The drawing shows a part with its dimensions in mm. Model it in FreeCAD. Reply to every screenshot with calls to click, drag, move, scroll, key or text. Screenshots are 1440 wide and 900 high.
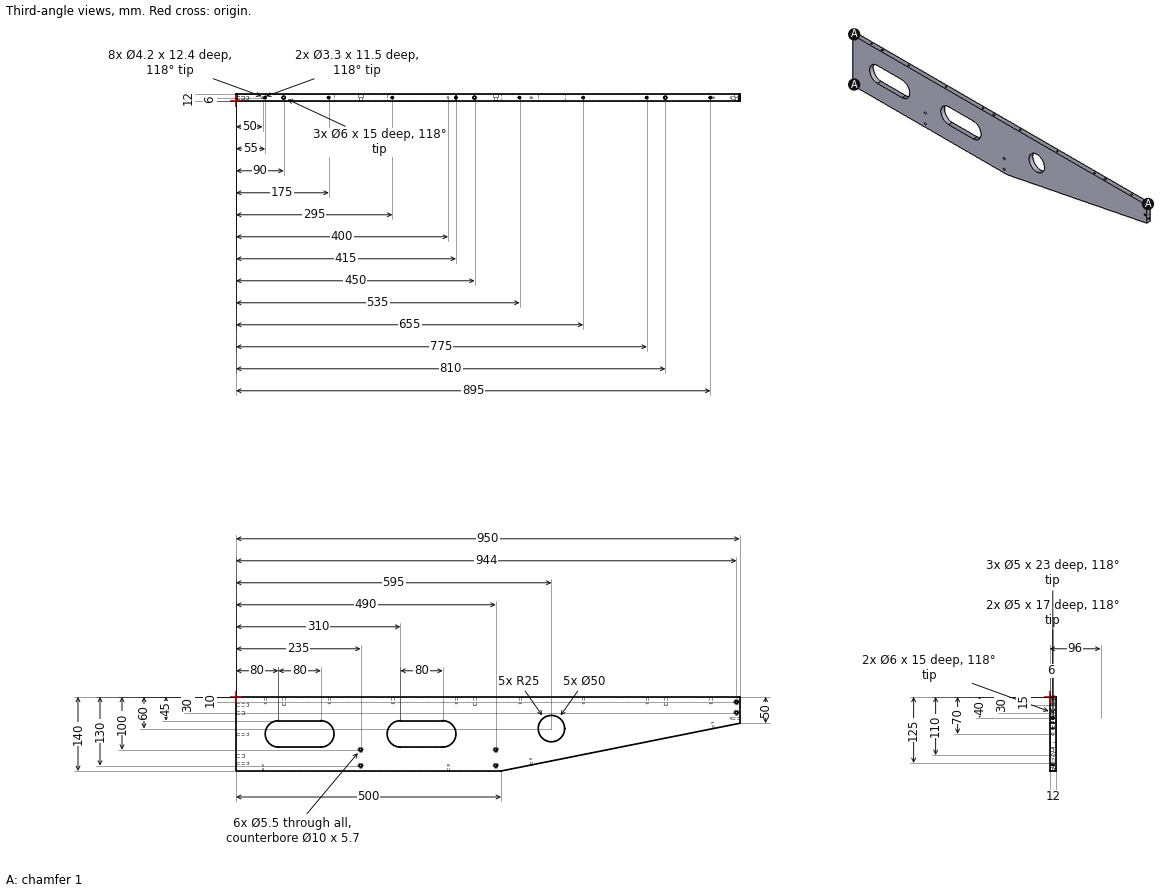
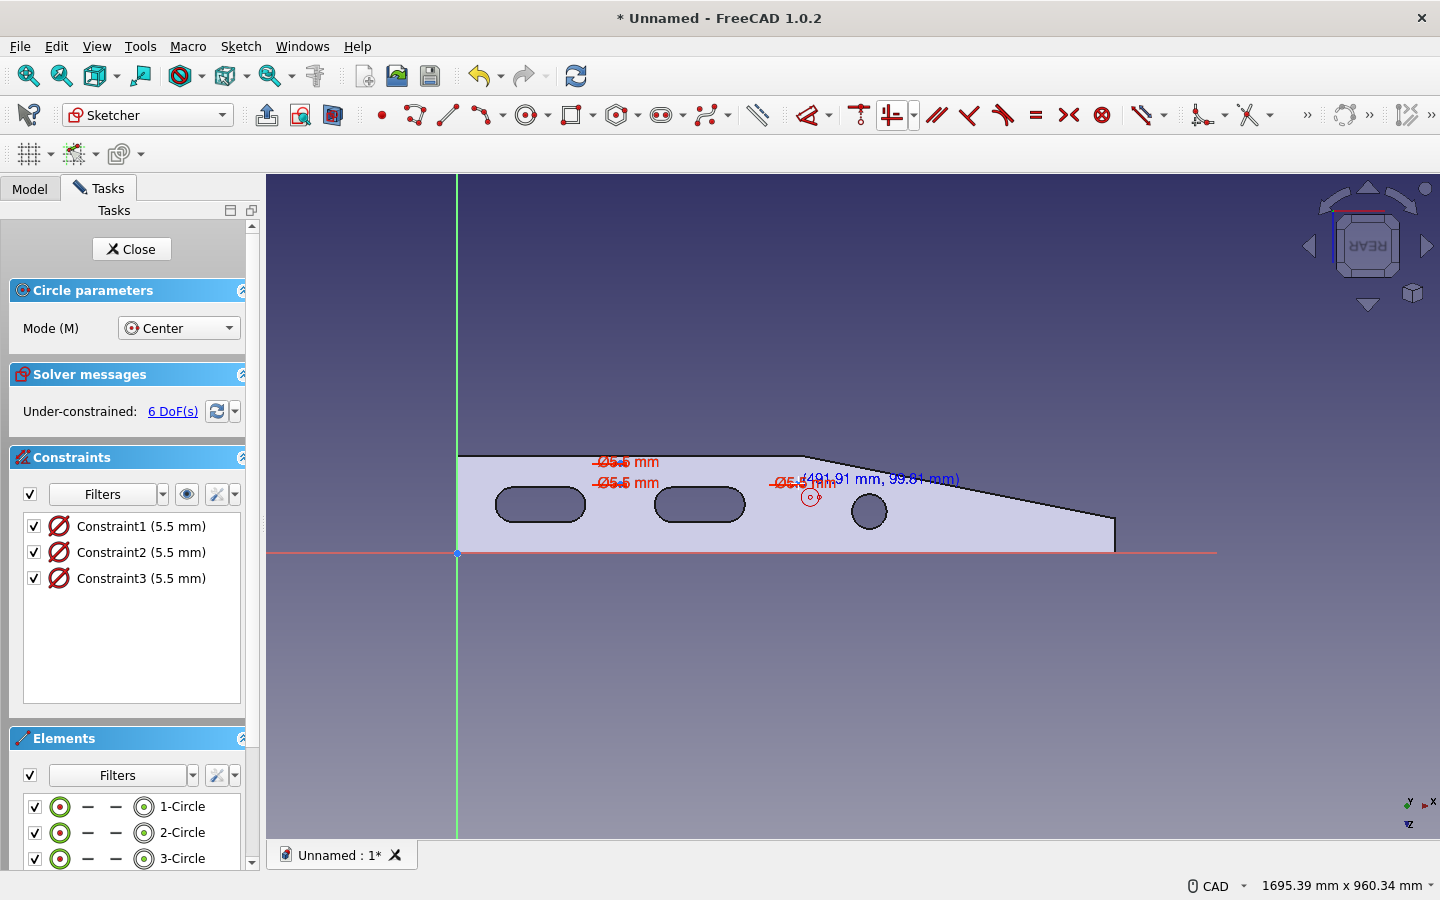
scroll(797, 463, up, 13)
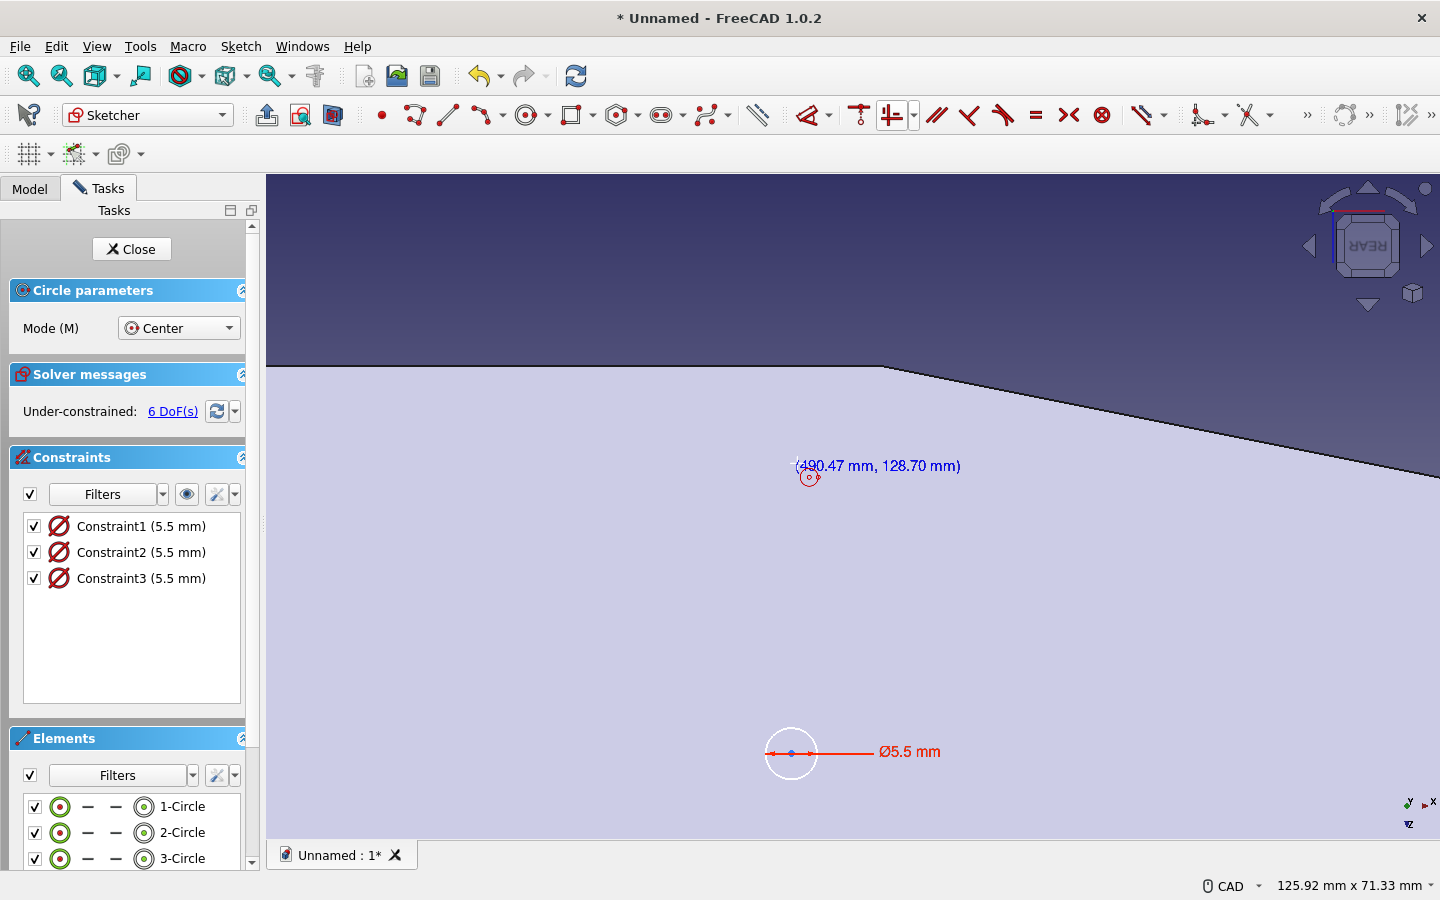
scroll(797, 463, down, 13)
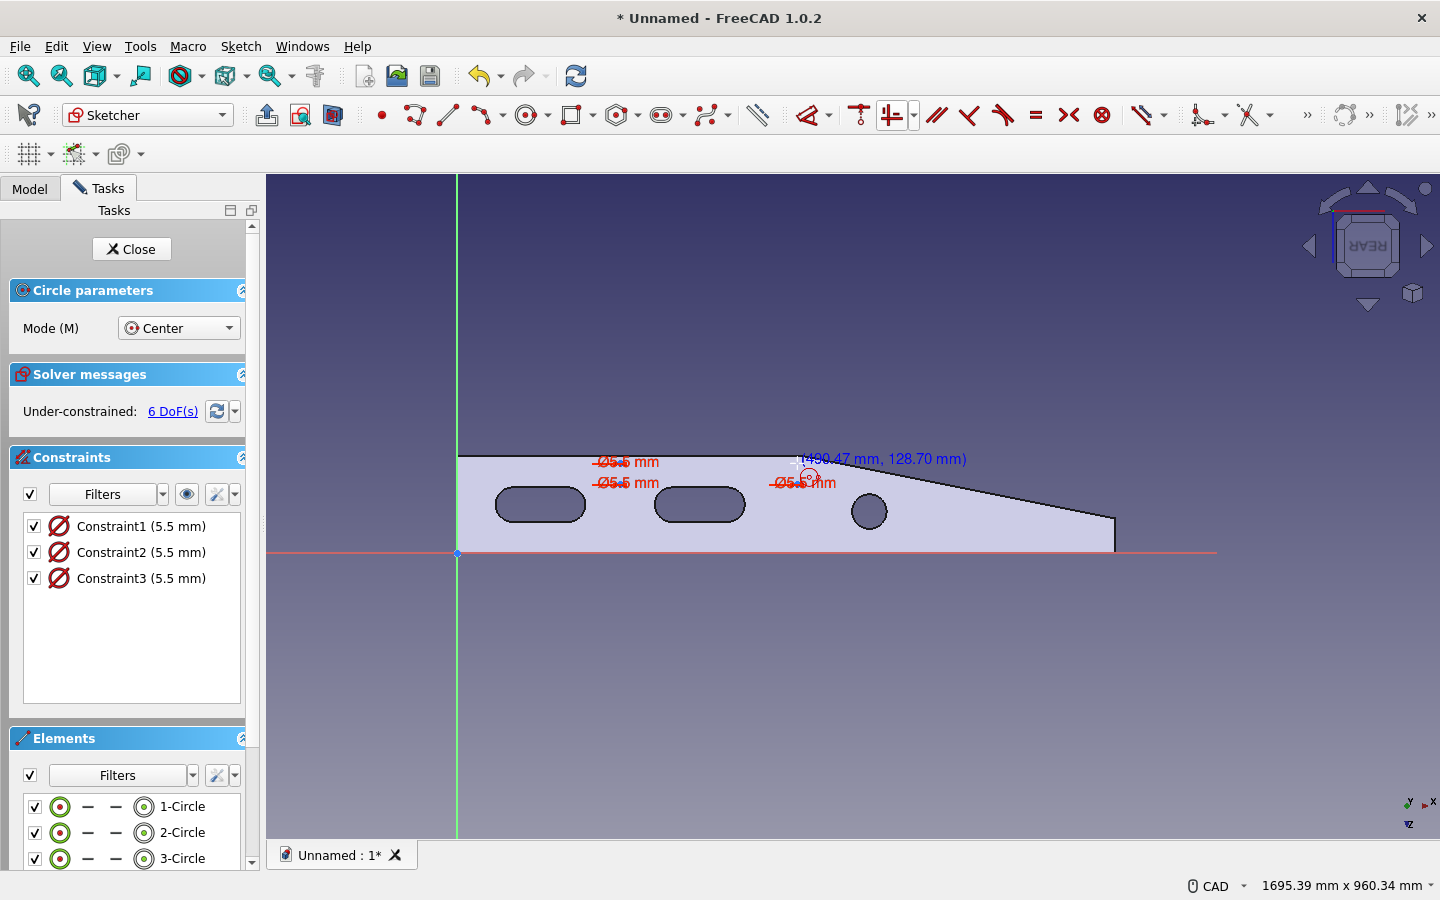
click(797, 463)
move(798, 462)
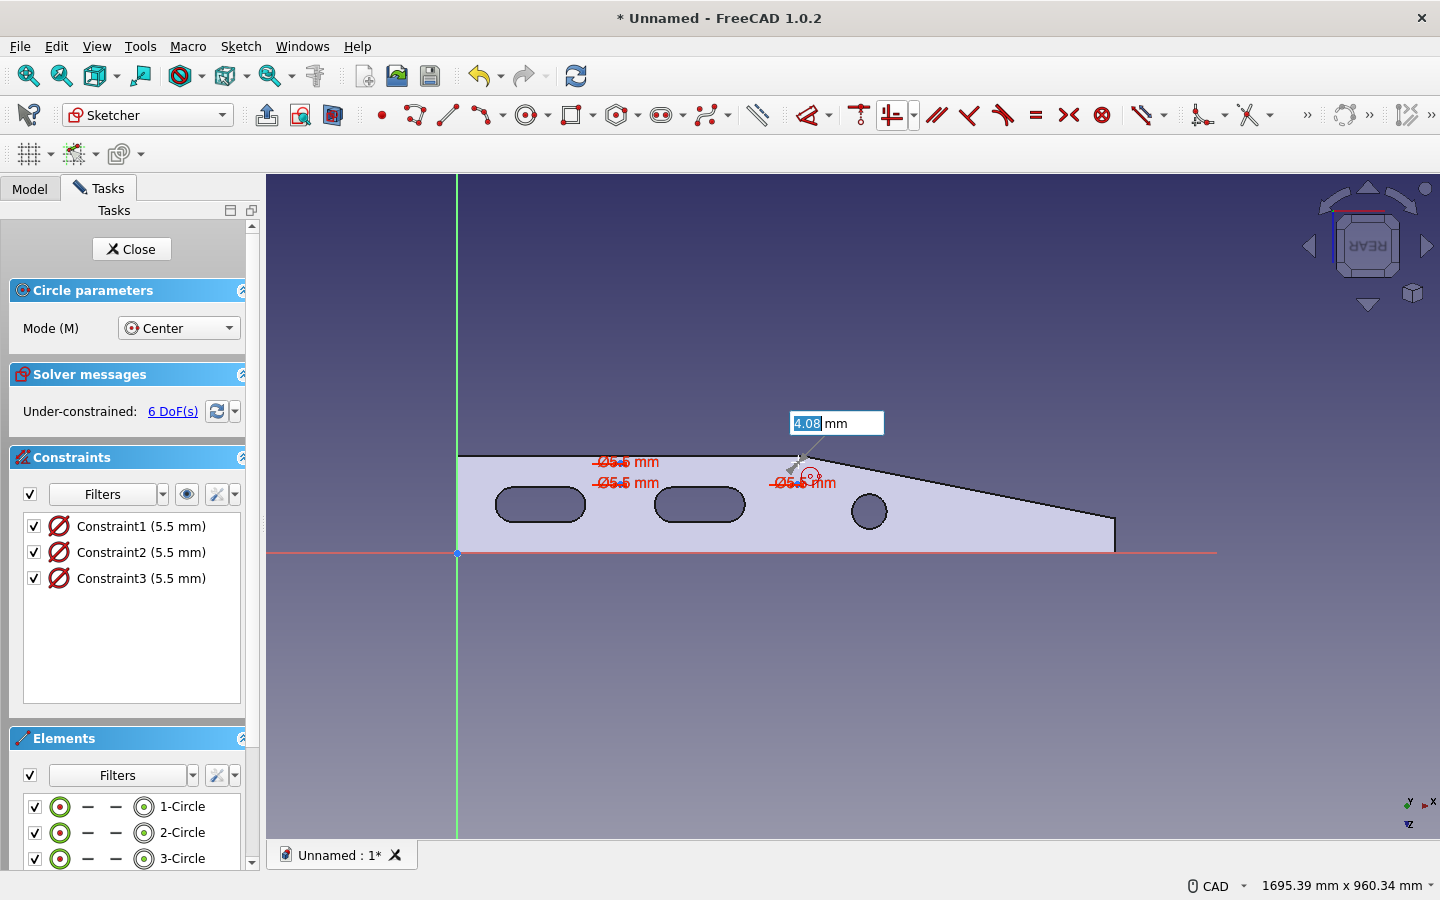
text(5.5)
key(Return)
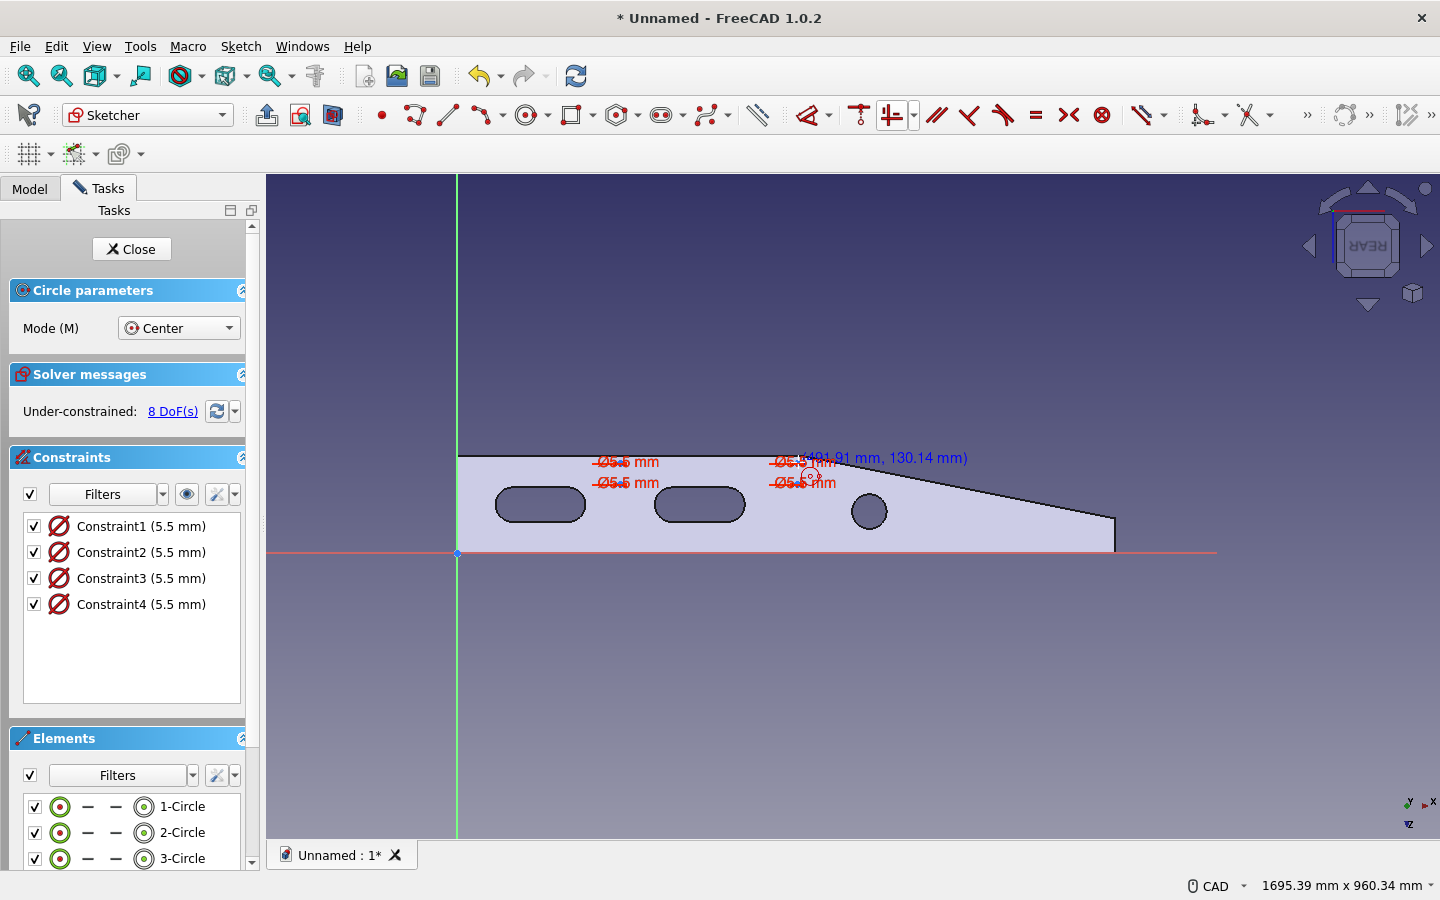
scroll(1111, 546, up, 13)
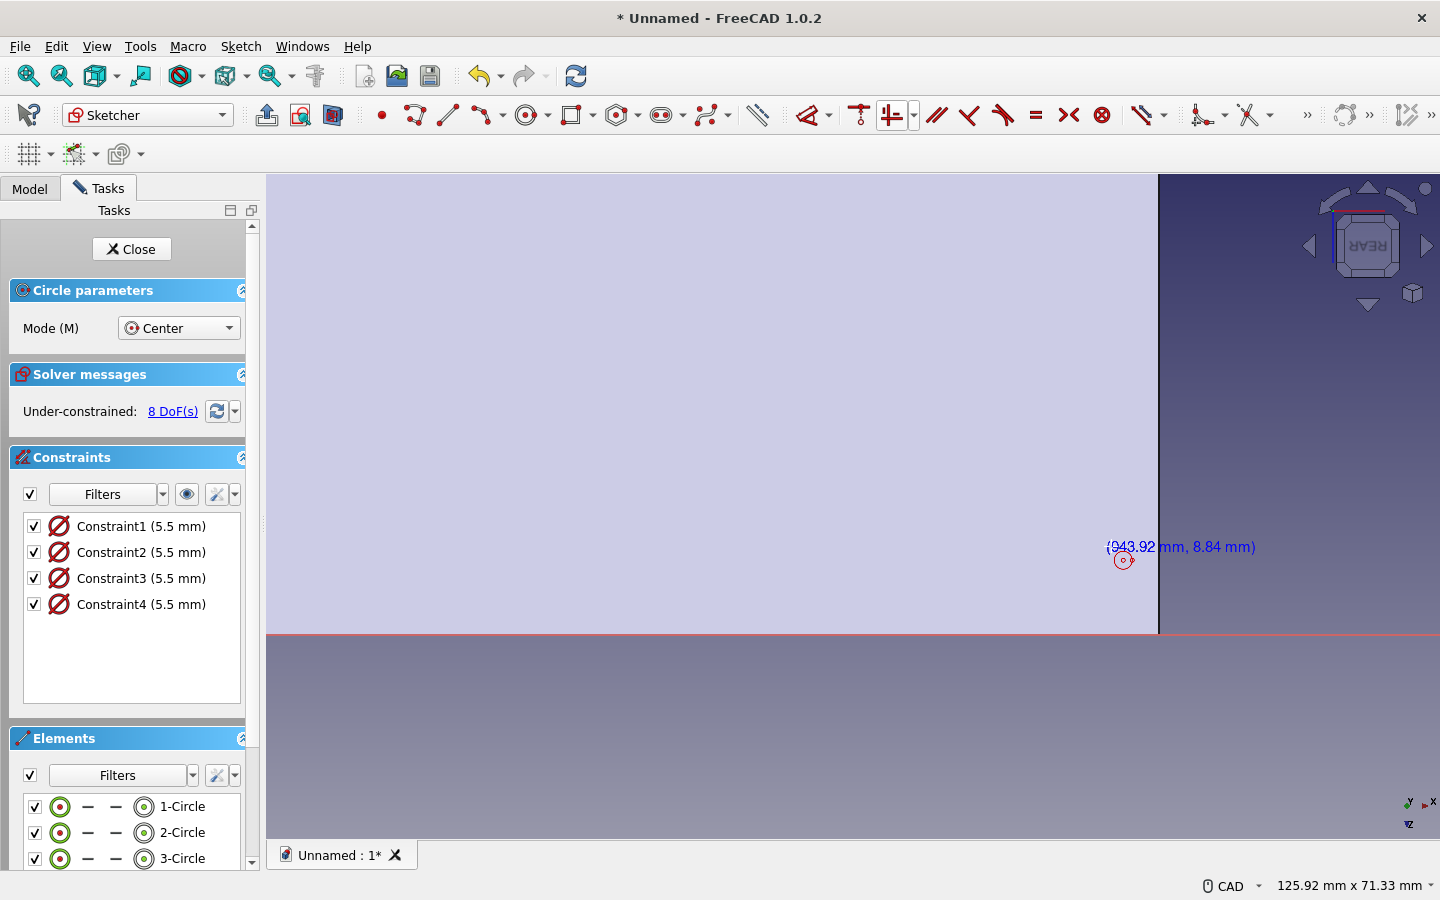
scroll(1111, 546, down, 13)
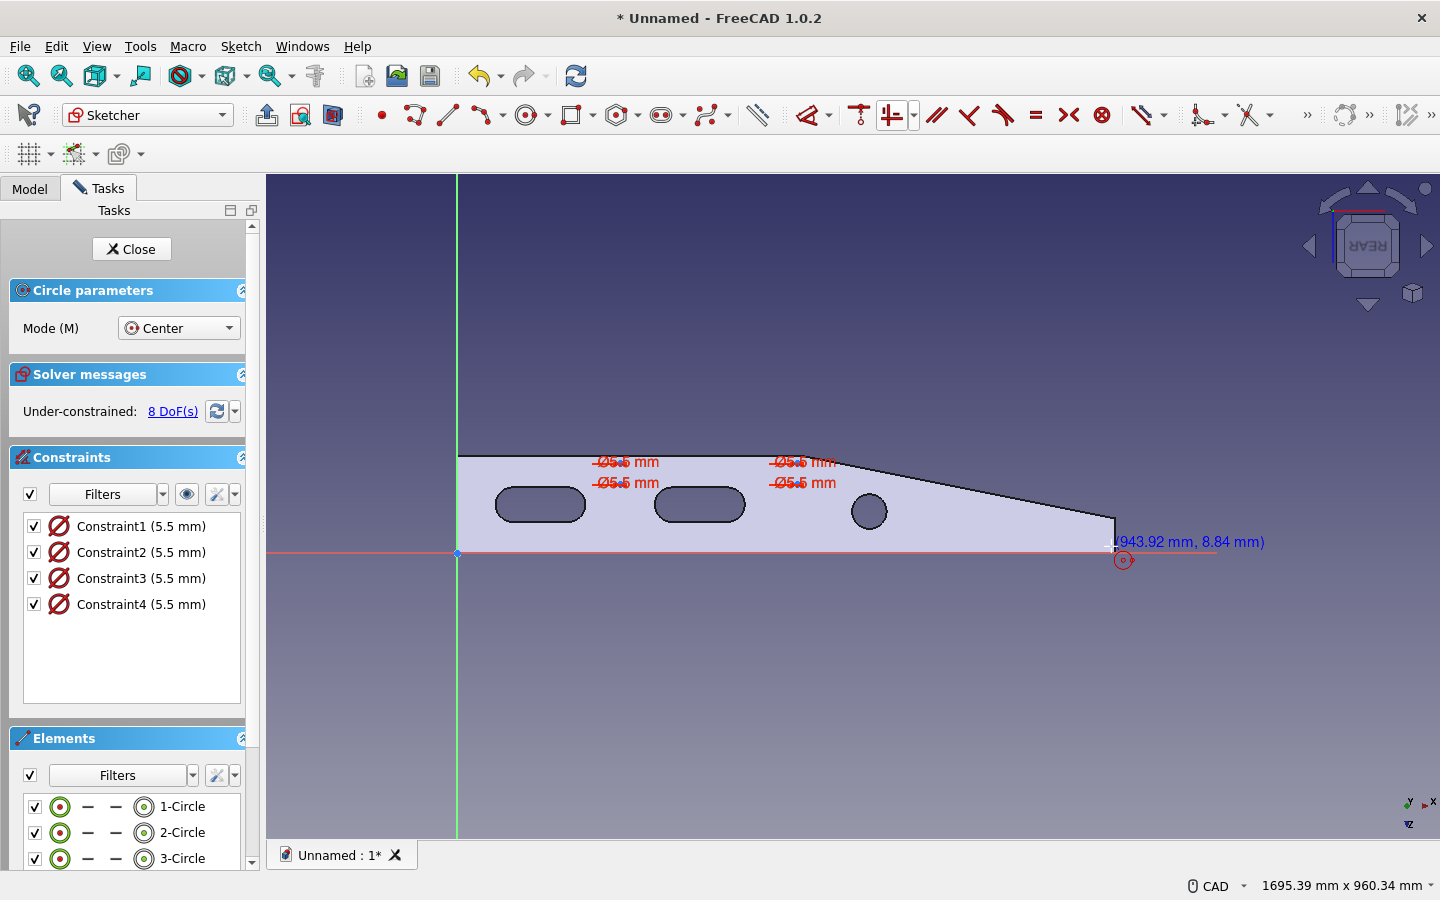
scroll(1111, 546, up, 5)